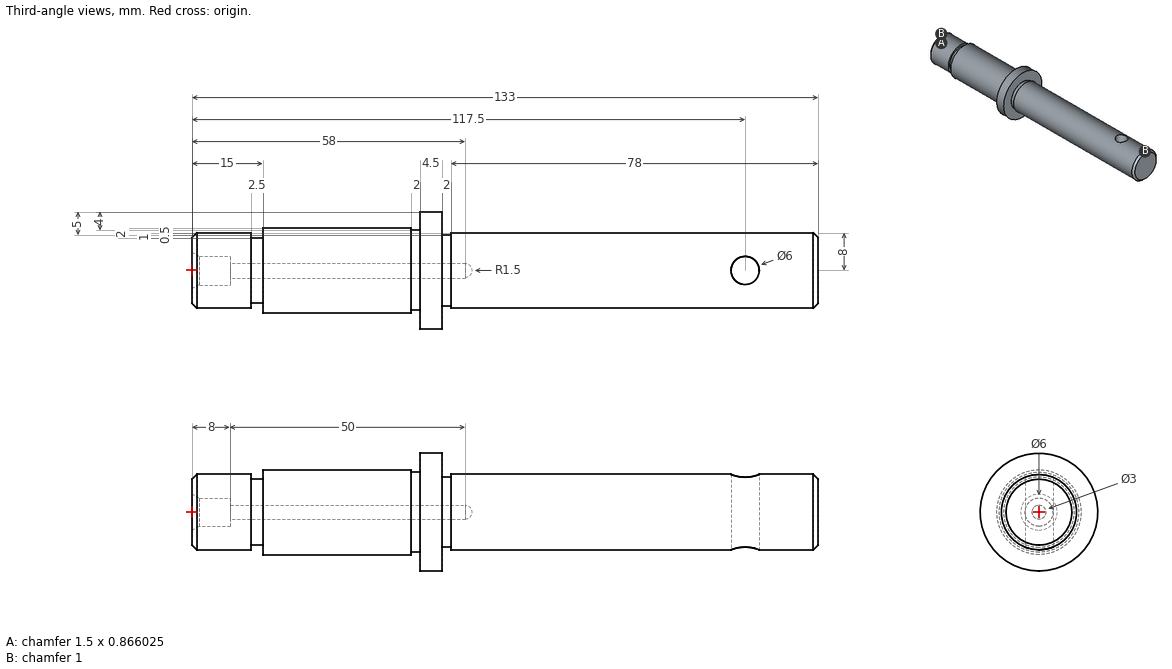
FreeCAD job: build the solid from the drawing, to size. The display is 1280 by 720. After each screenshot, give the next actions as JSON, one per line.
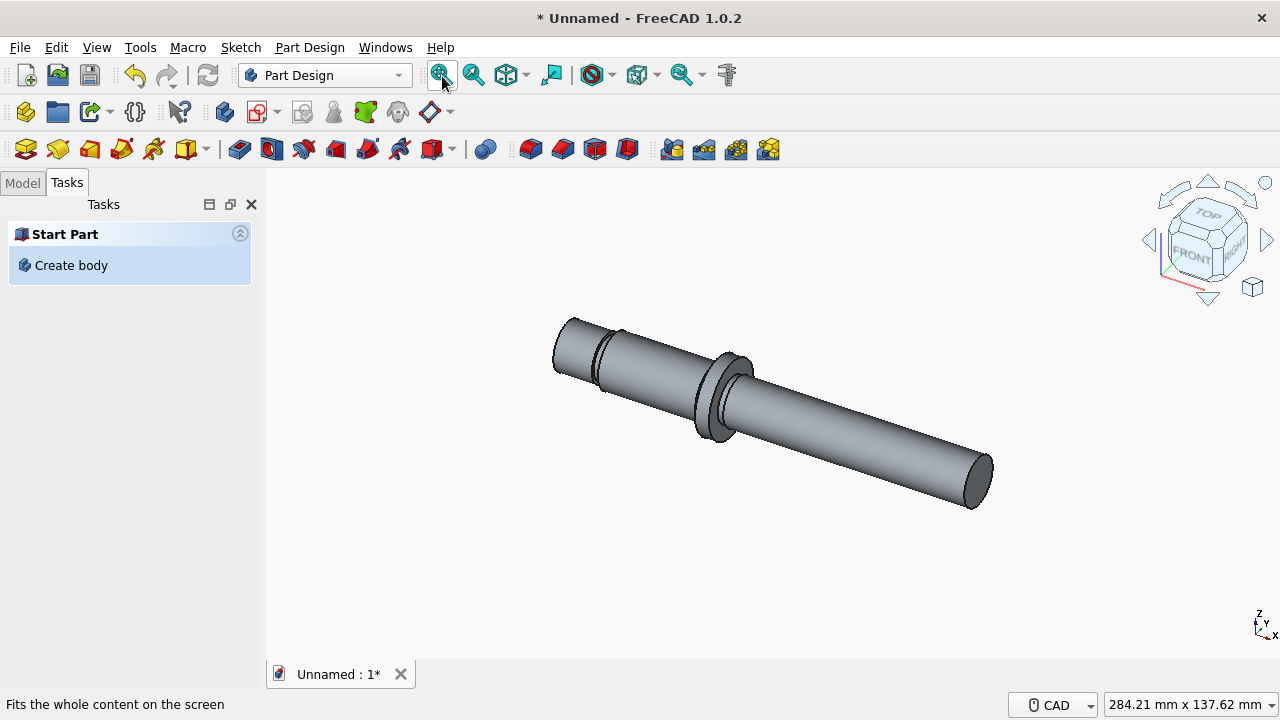
{"action": "left_click", "coordinate": [258, 112]}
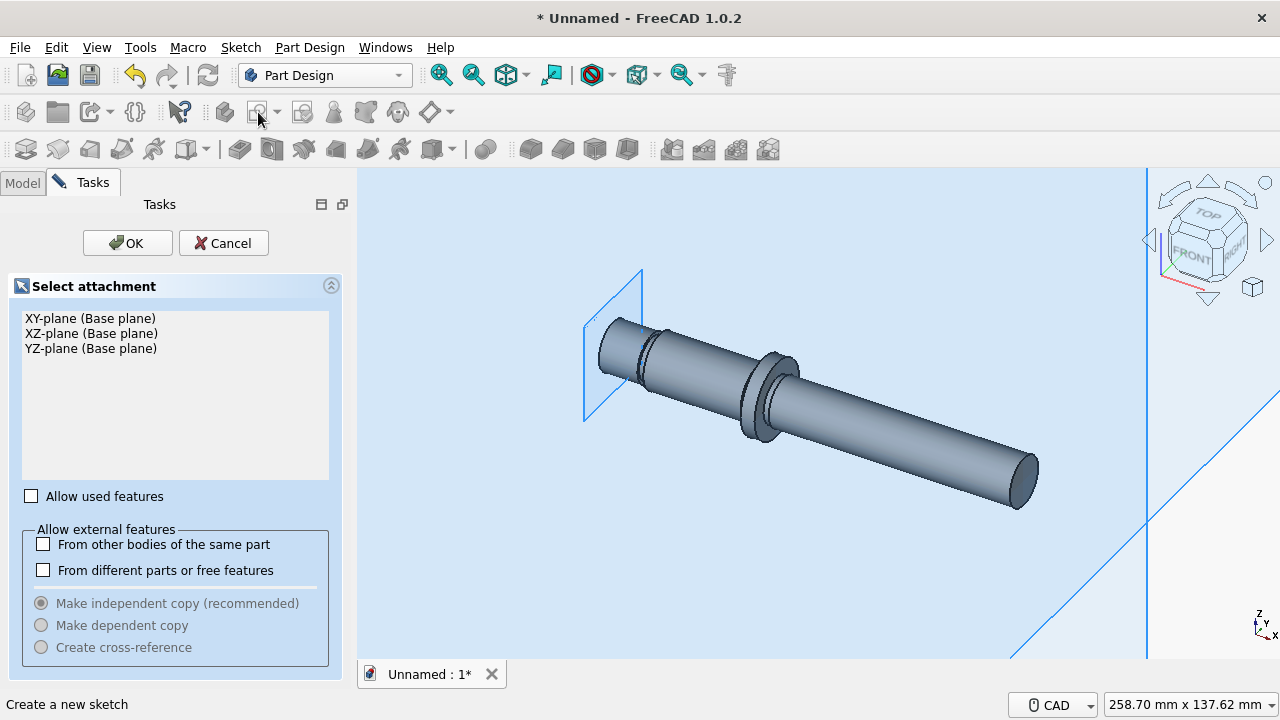
{"action": "left_click", "coordinate": [82, 318]}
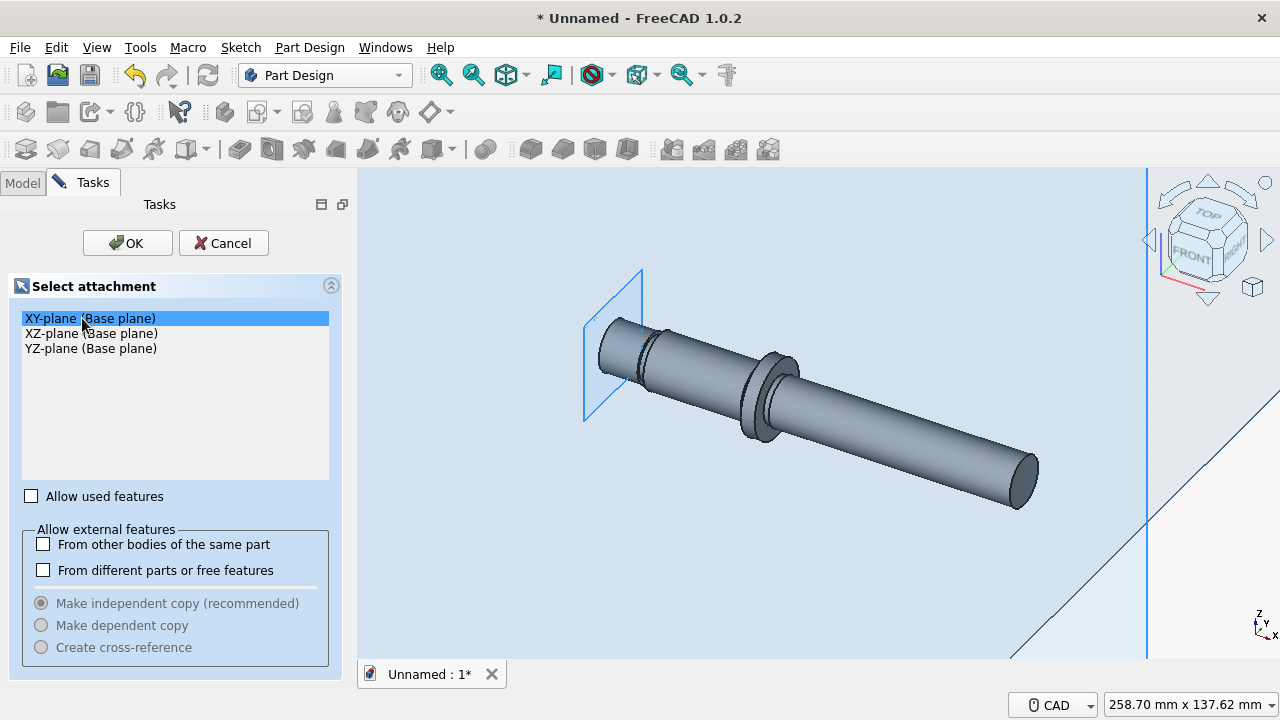
{"action": "left_click", "coordinate": [128, 243]}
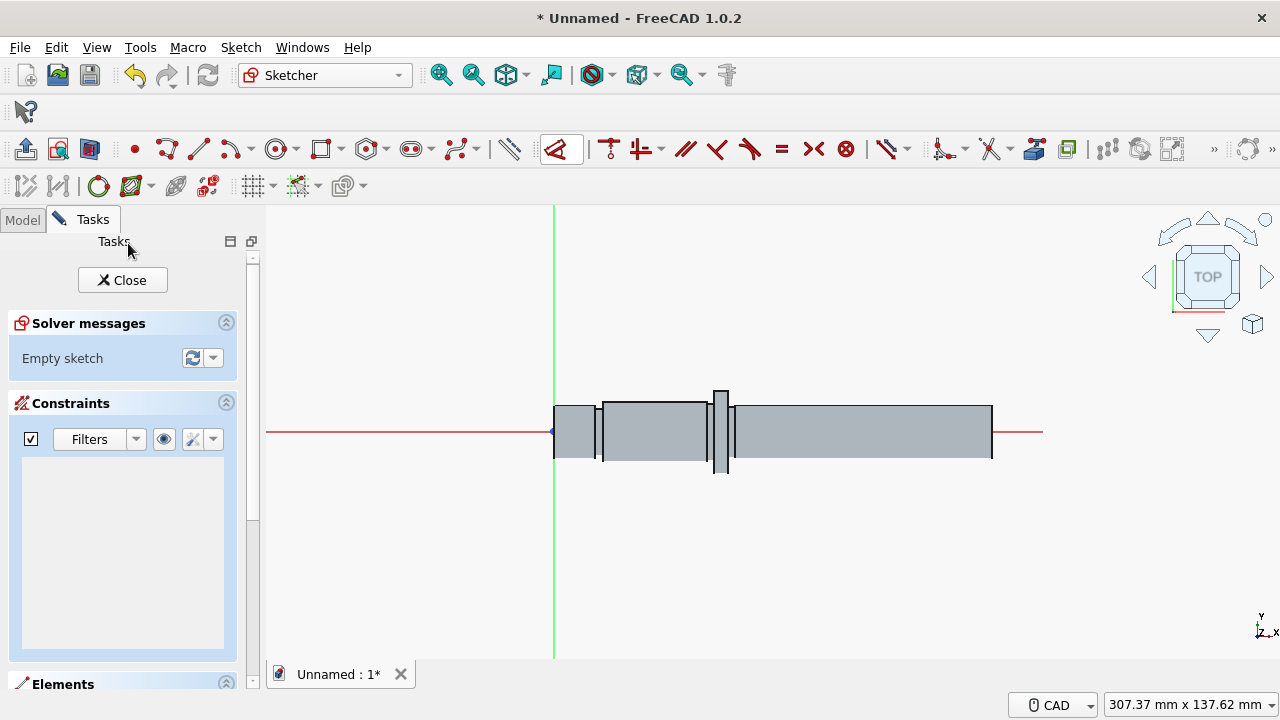
{"action": "left_click", "coordinate": [90, 150]}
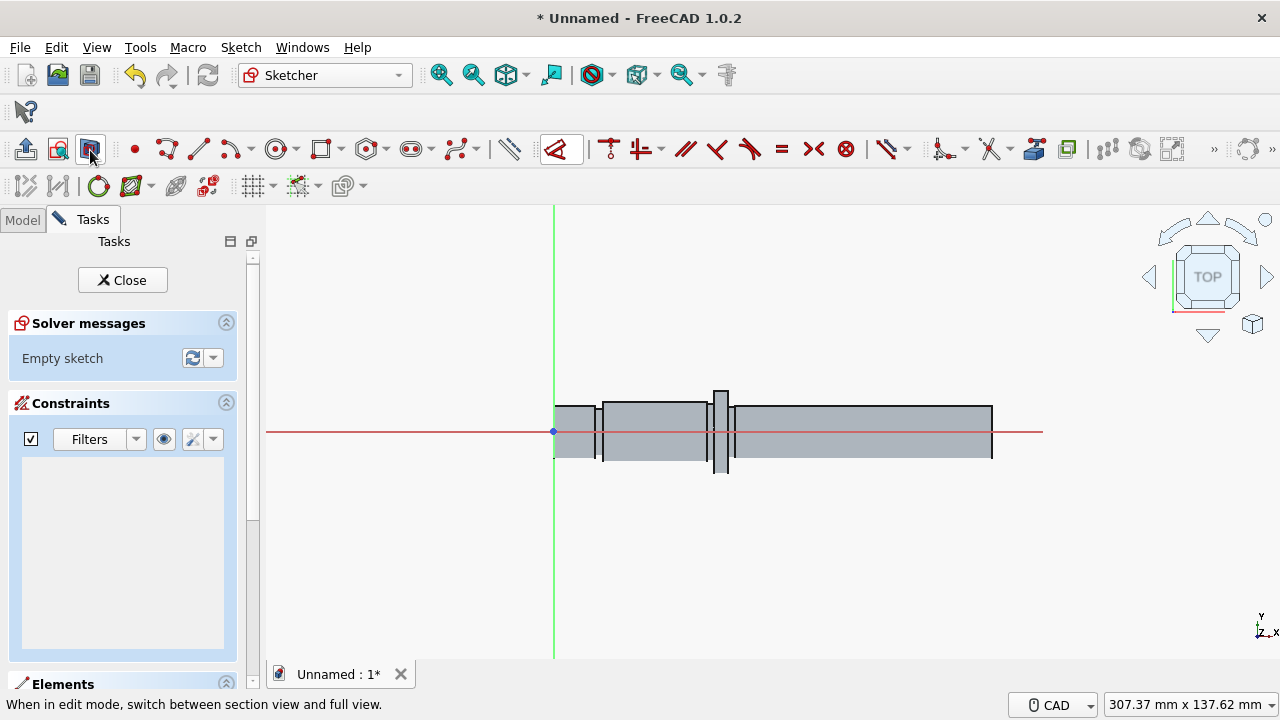
{"action": "scroll", "coordinate": [960, 432], "scroll_direction": "up", "scroll_amount": 13}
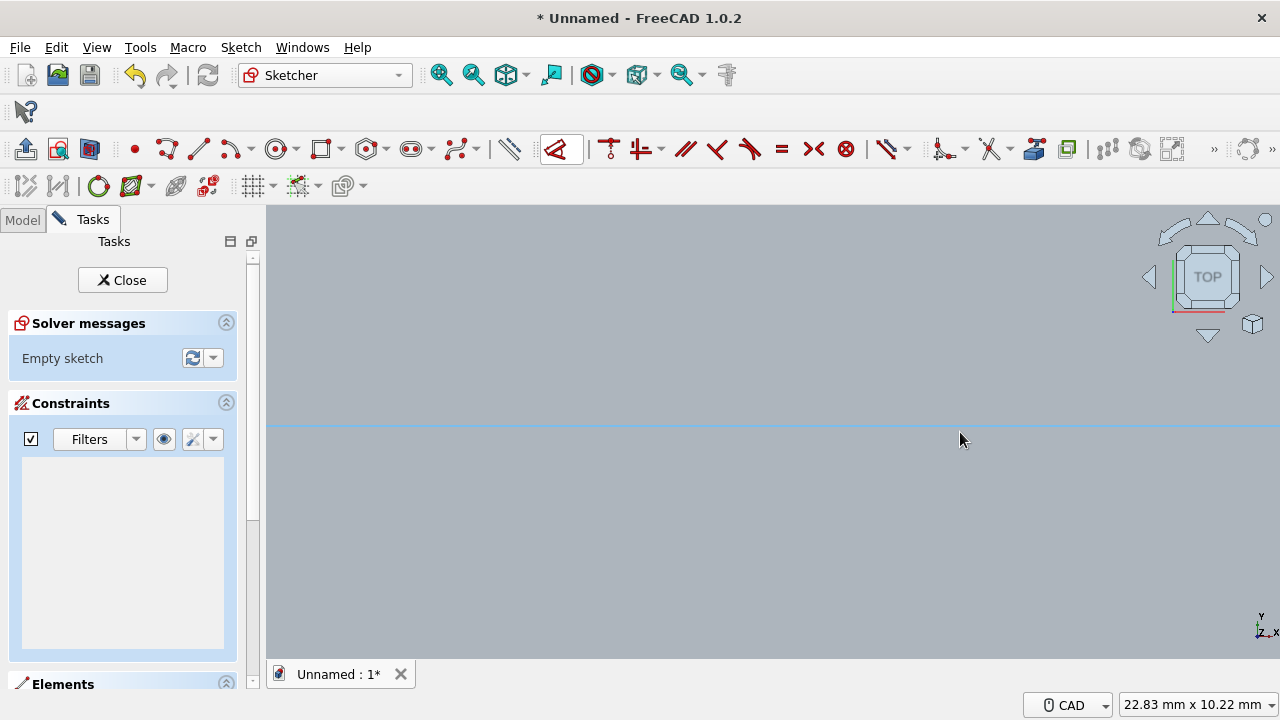
{"action": "key", "text": "g c"}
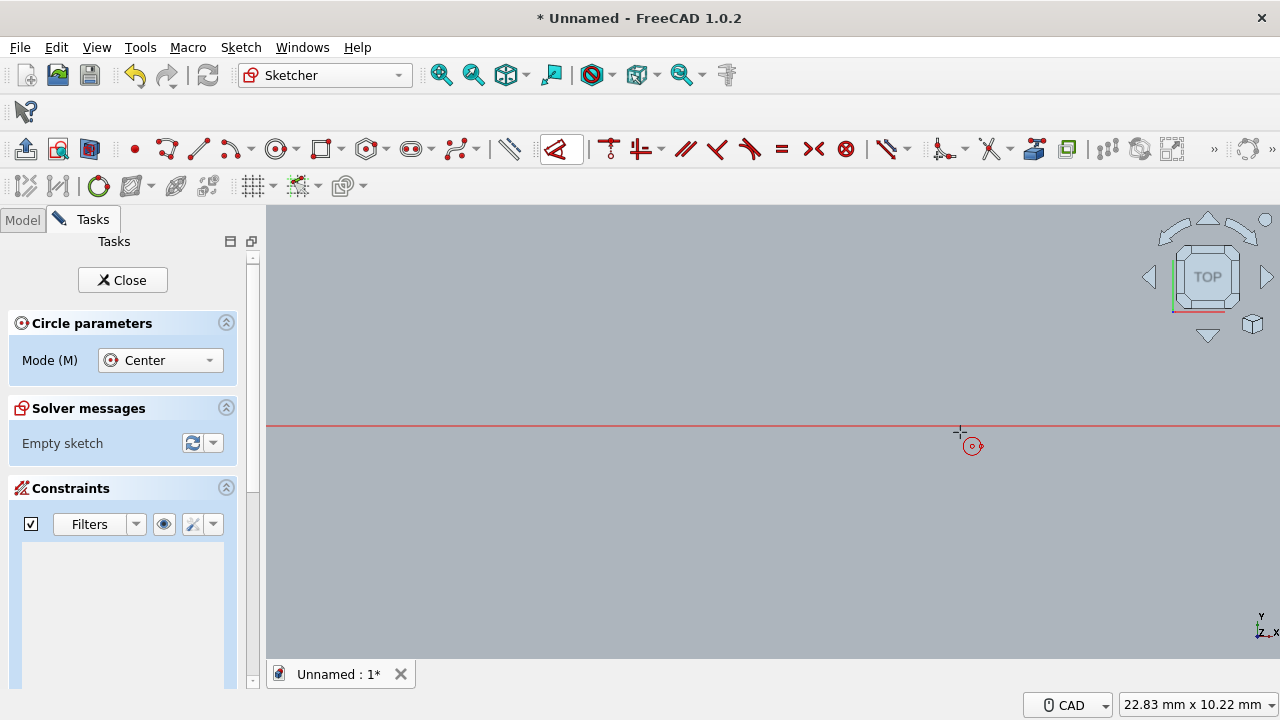
{"action": "left_click", "coordinate": [699, 426]}
{"action": "mouse_move", "coordinate": [793, 332]}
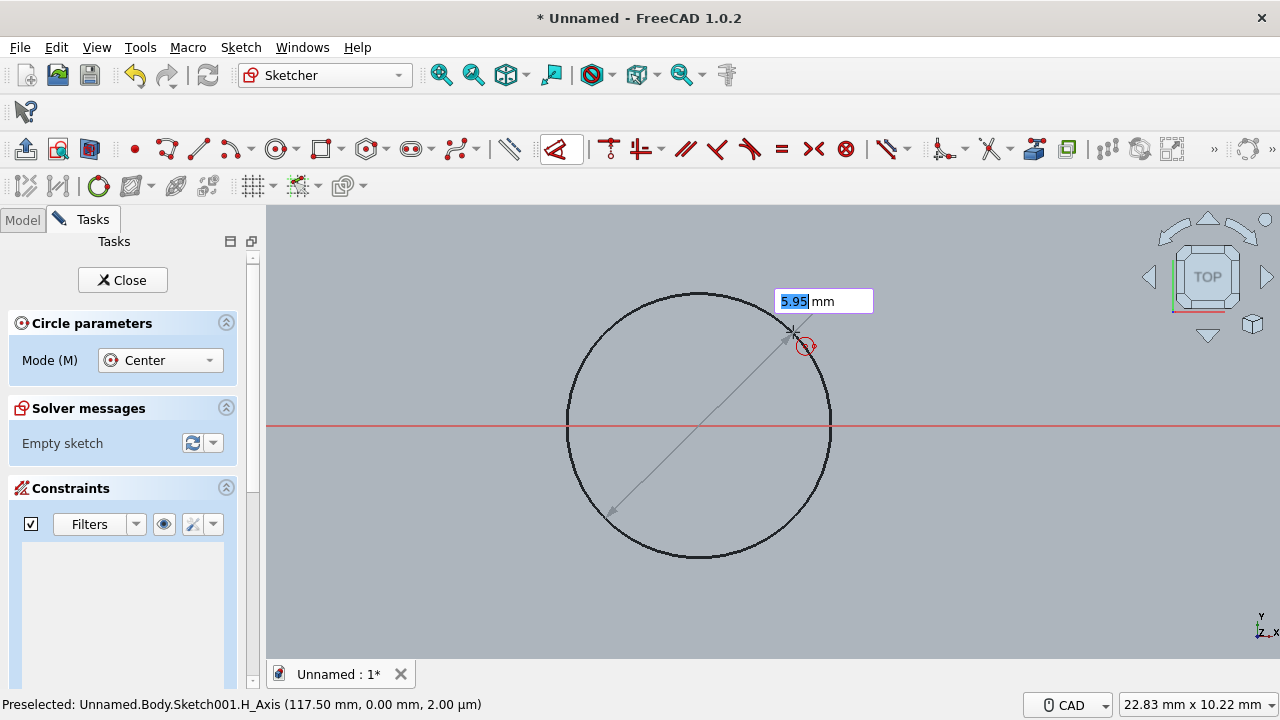
{"action": "type", "text": "6"}
{"action": "key", "text": "Return"}
{"action": "key", "text": "Escape"}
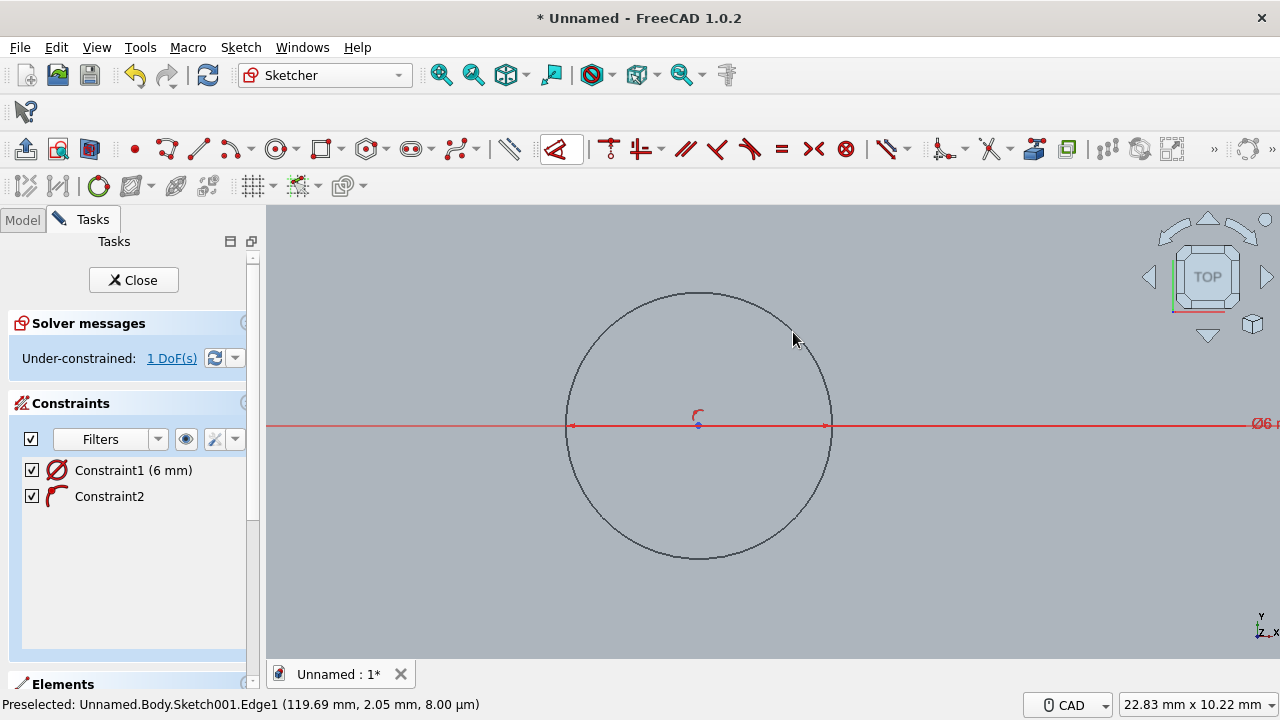
{"action": "left_click", "coordinate": [699, 426]}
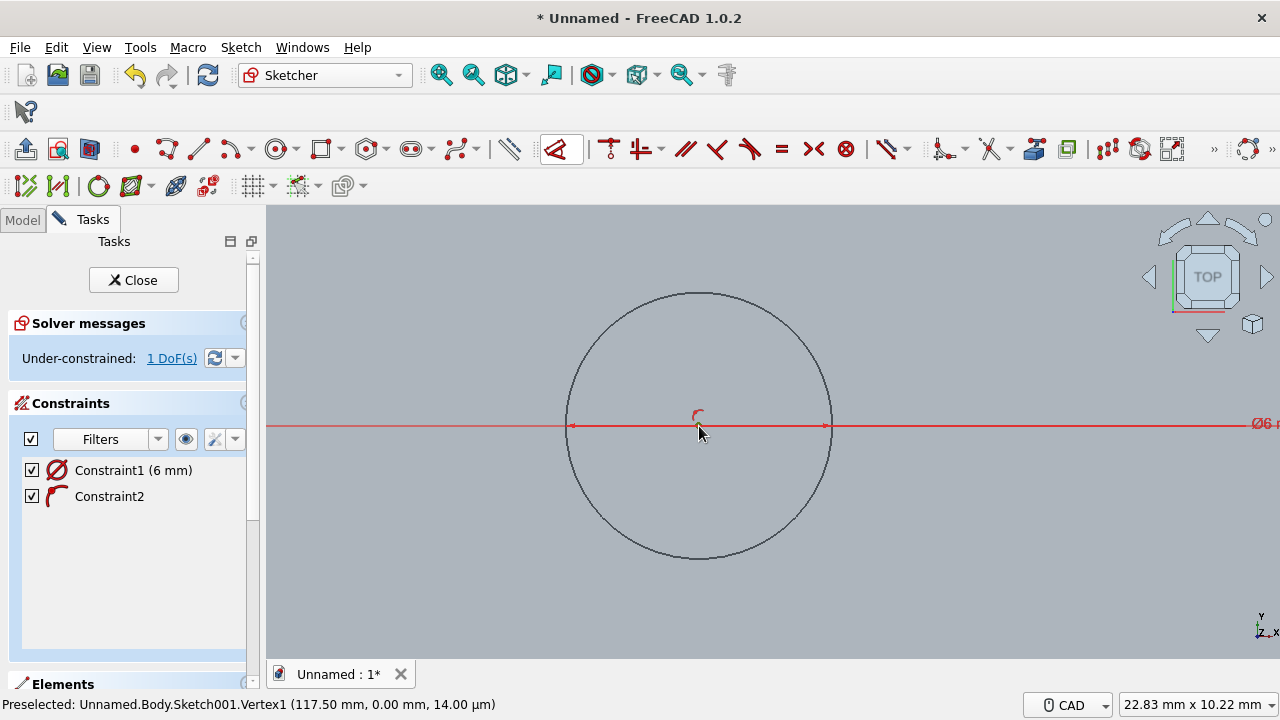
{"action": "key", "text": "l"}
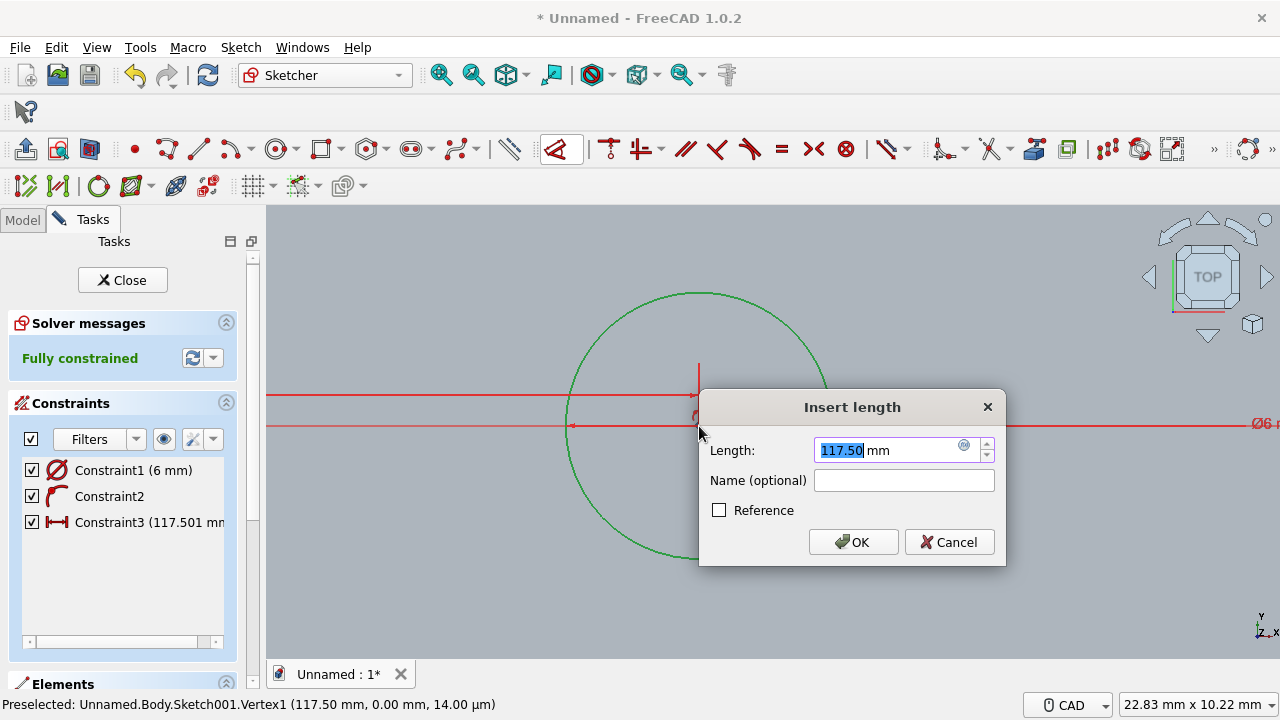
{"action": "type", "text": "117.5"}
{"action": "key", "text": "Return"}